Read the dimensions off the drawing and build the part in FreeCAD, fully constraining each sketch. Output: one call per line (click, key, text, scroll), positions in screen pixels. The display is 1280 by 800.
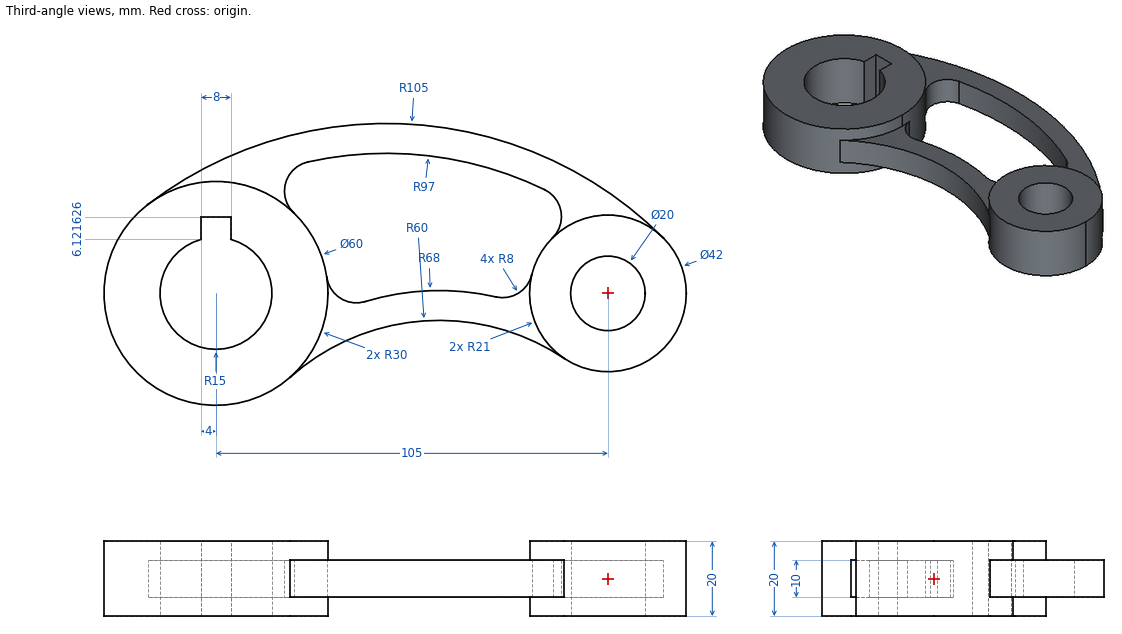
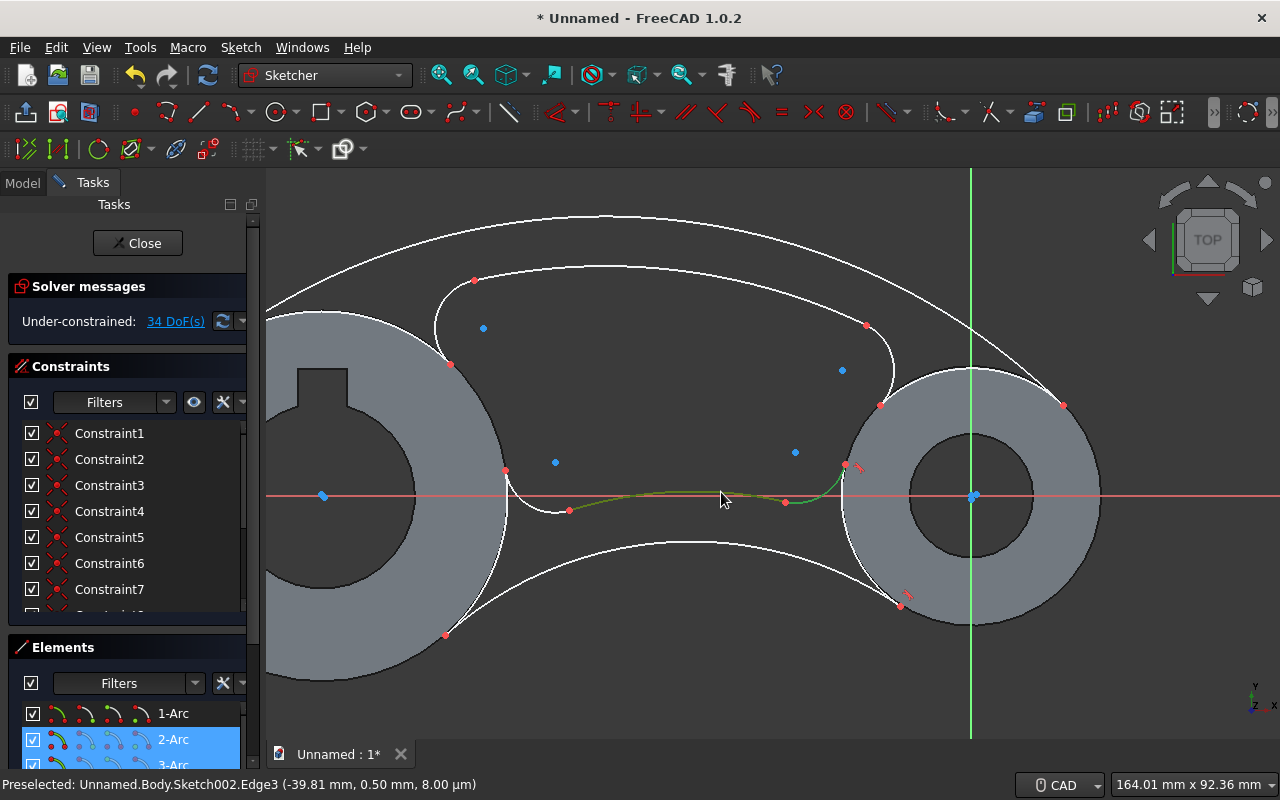
key(t)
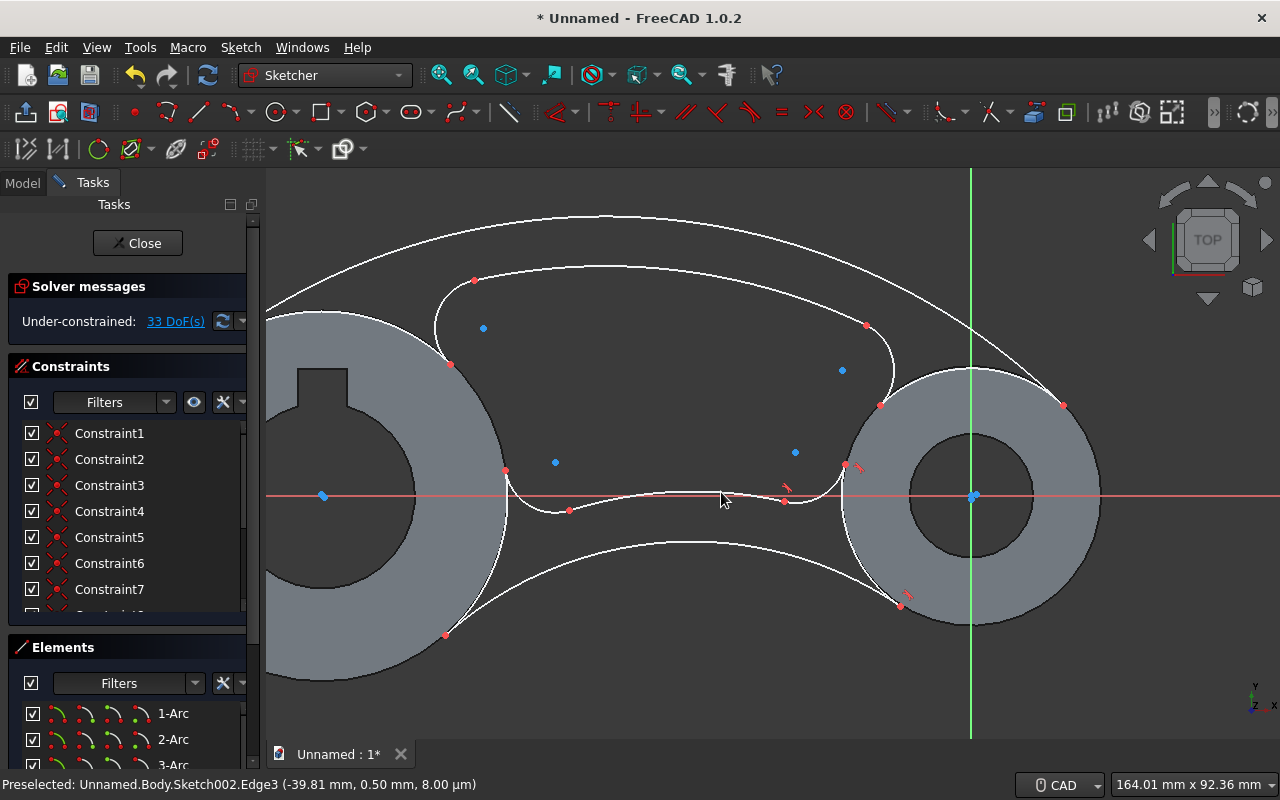
click(720, 492)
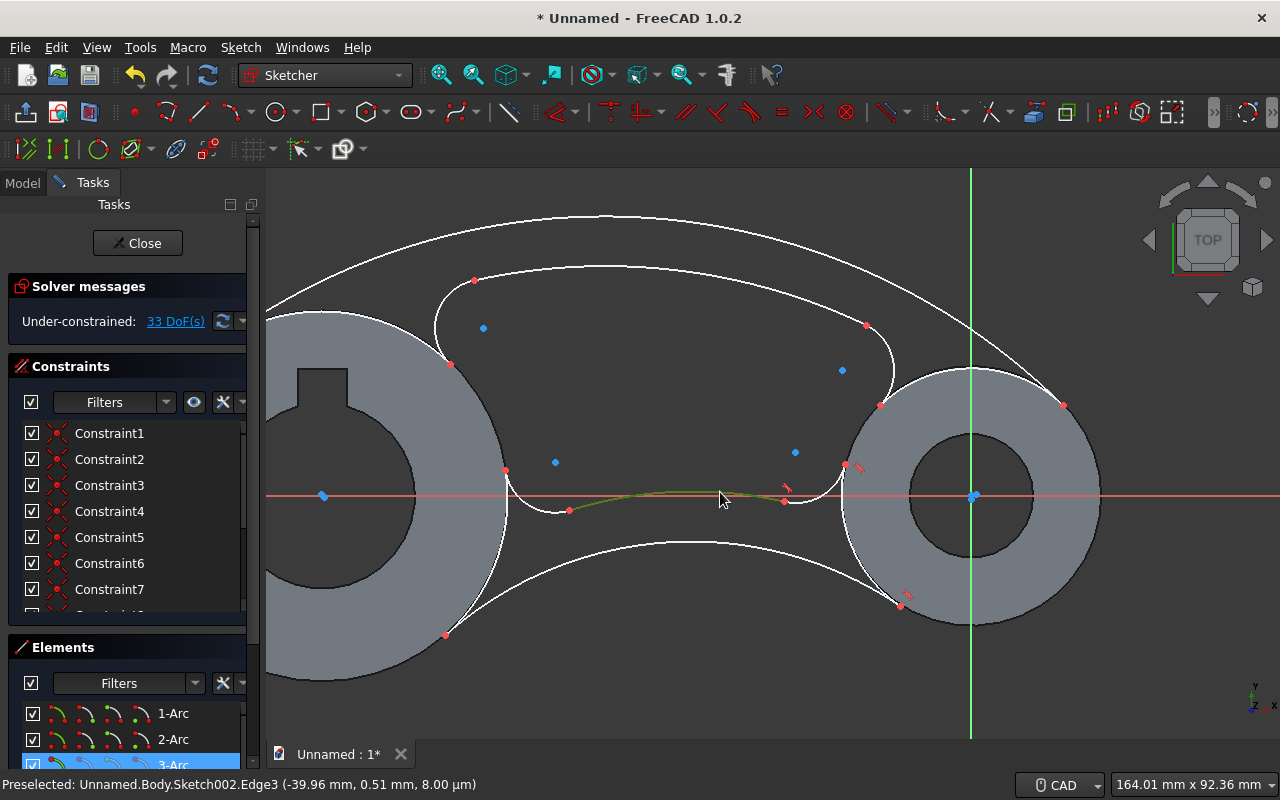
click(544, 511)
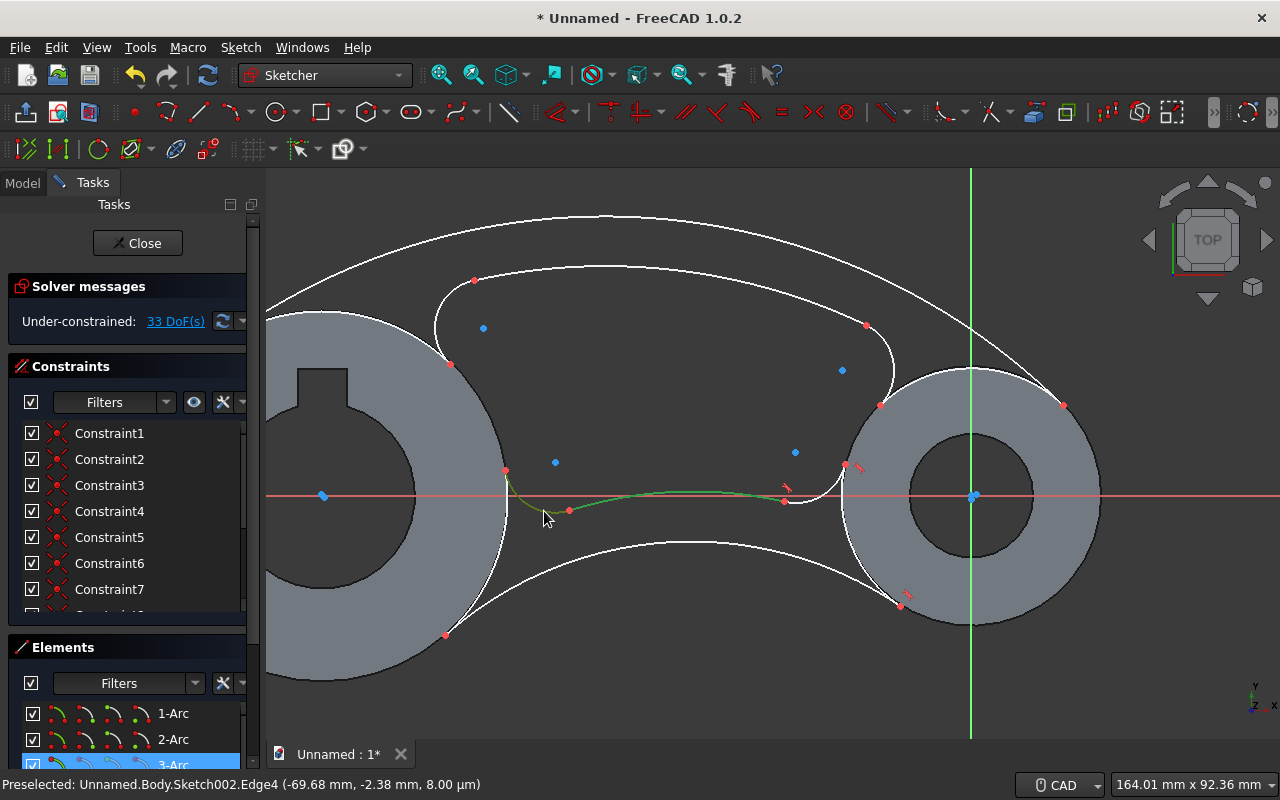
key(t)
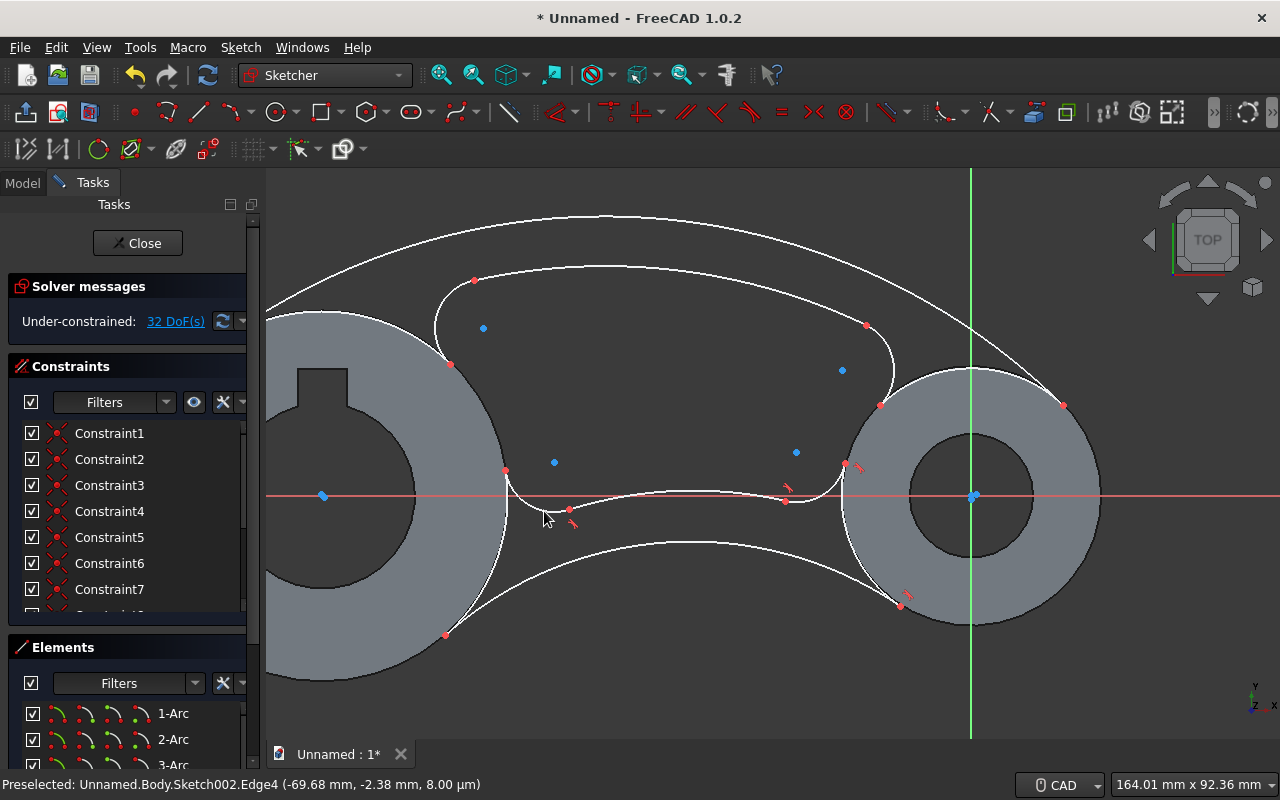
click(544, 511)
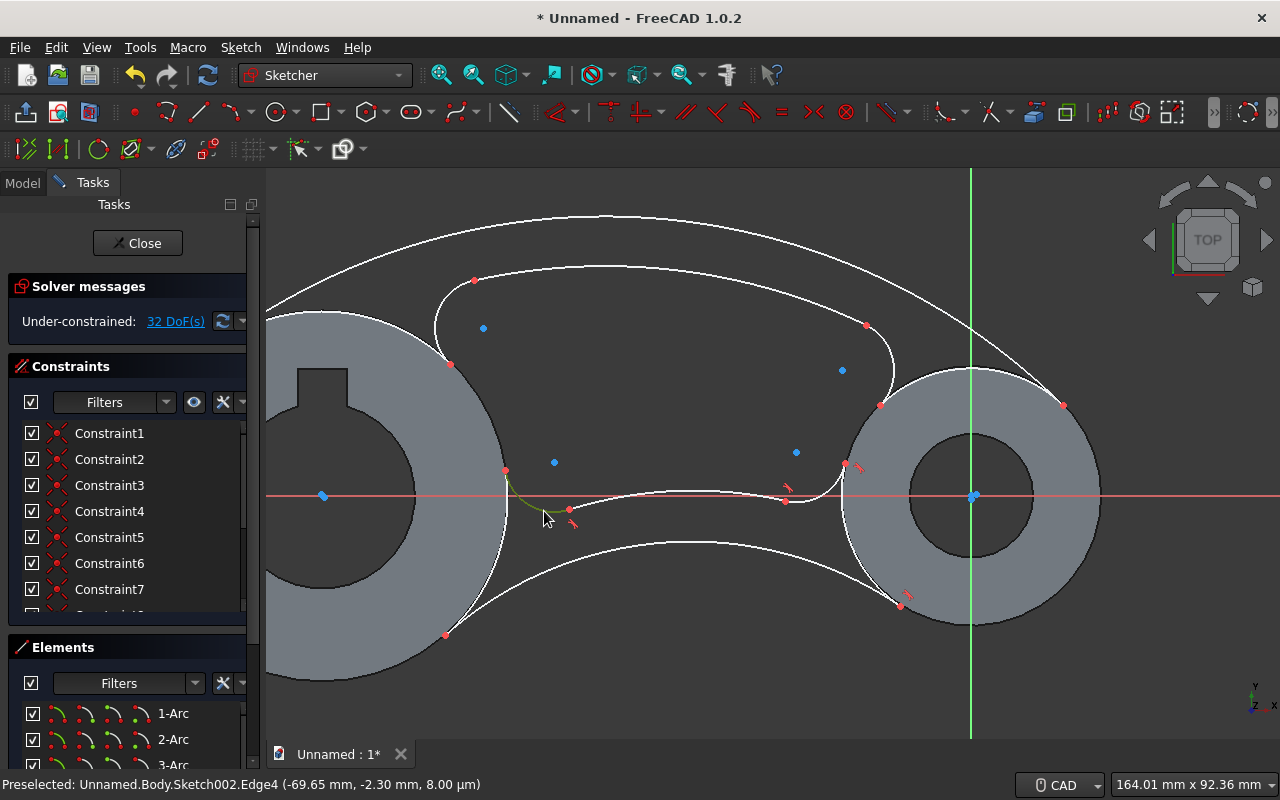
click(481, 593)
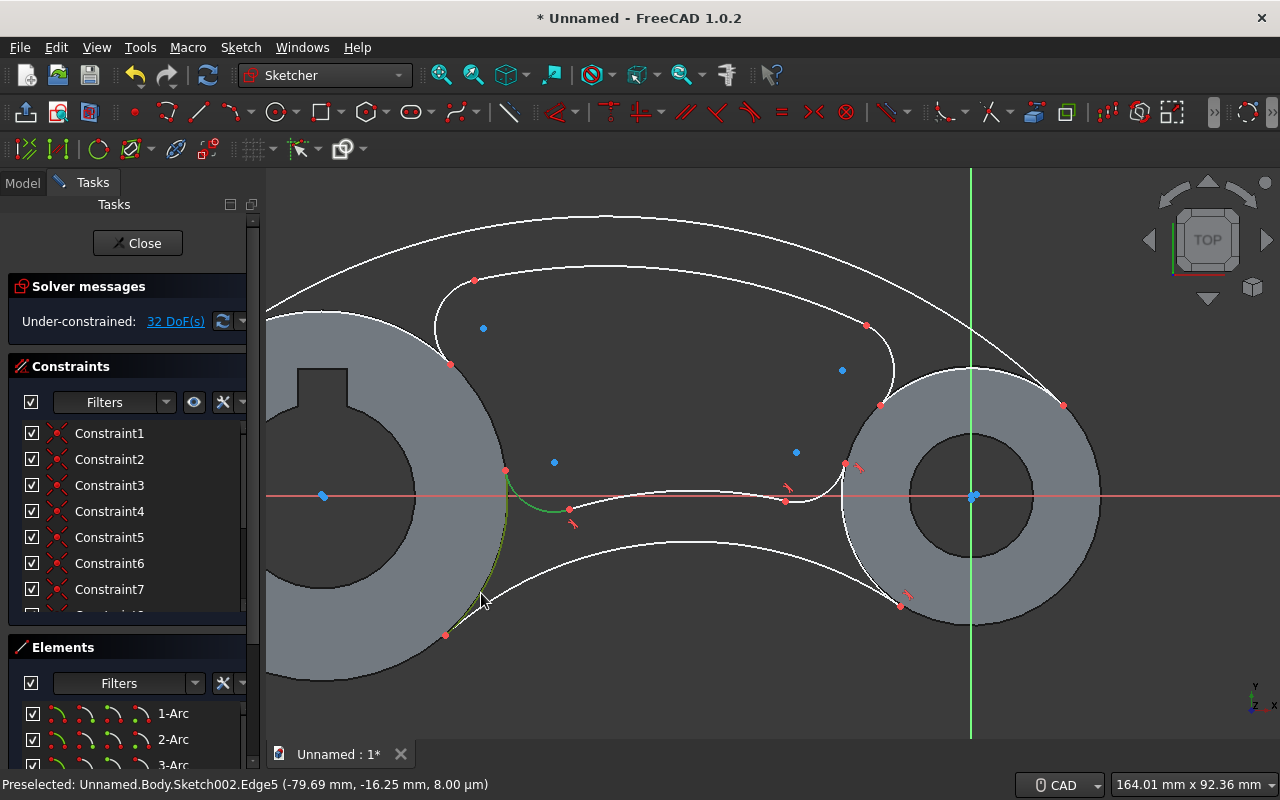
key(t)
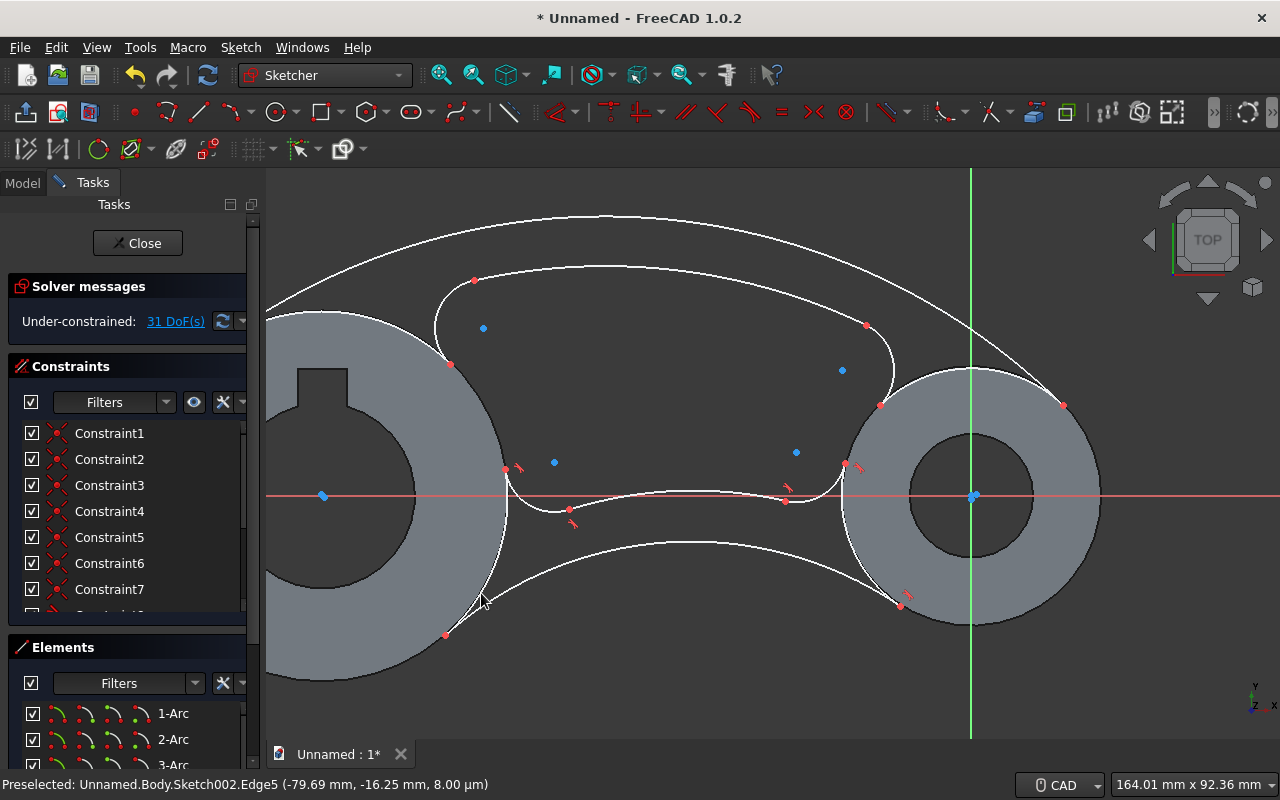
click(481, 593)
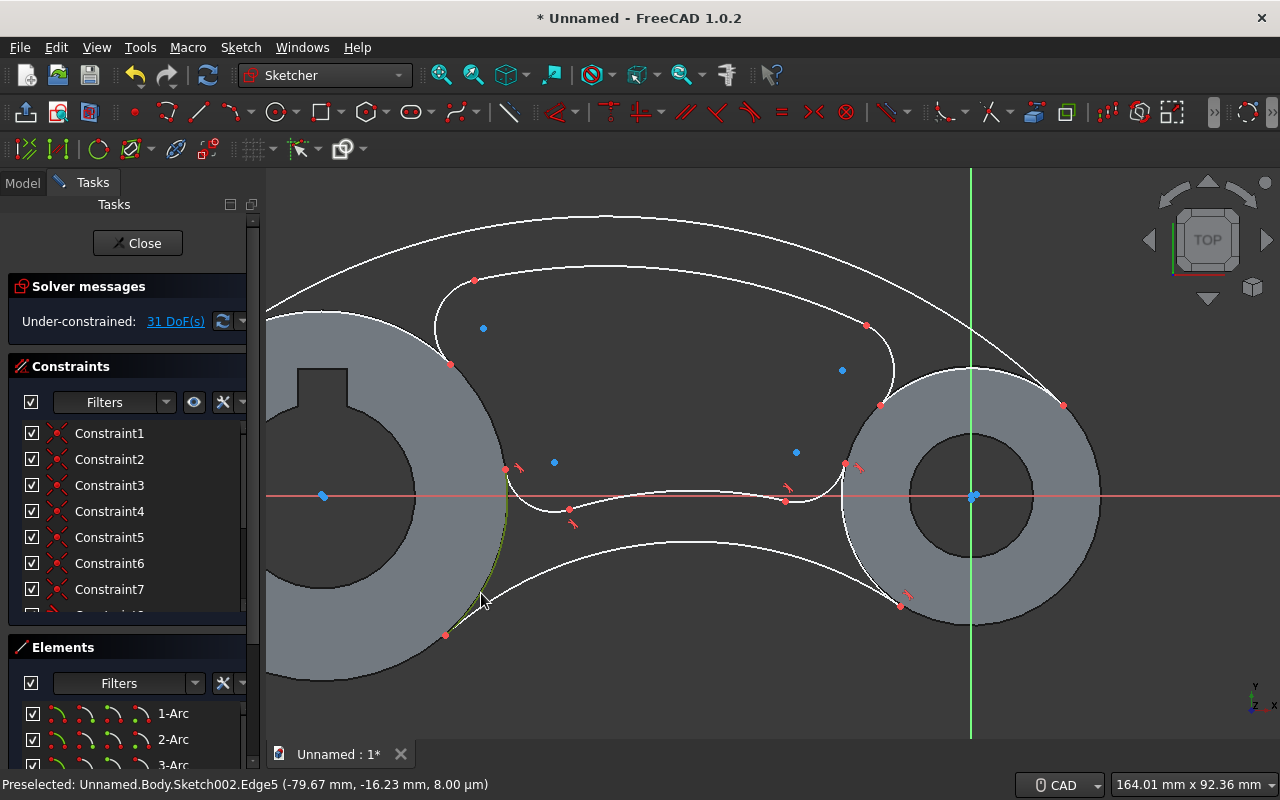
click(766, 549)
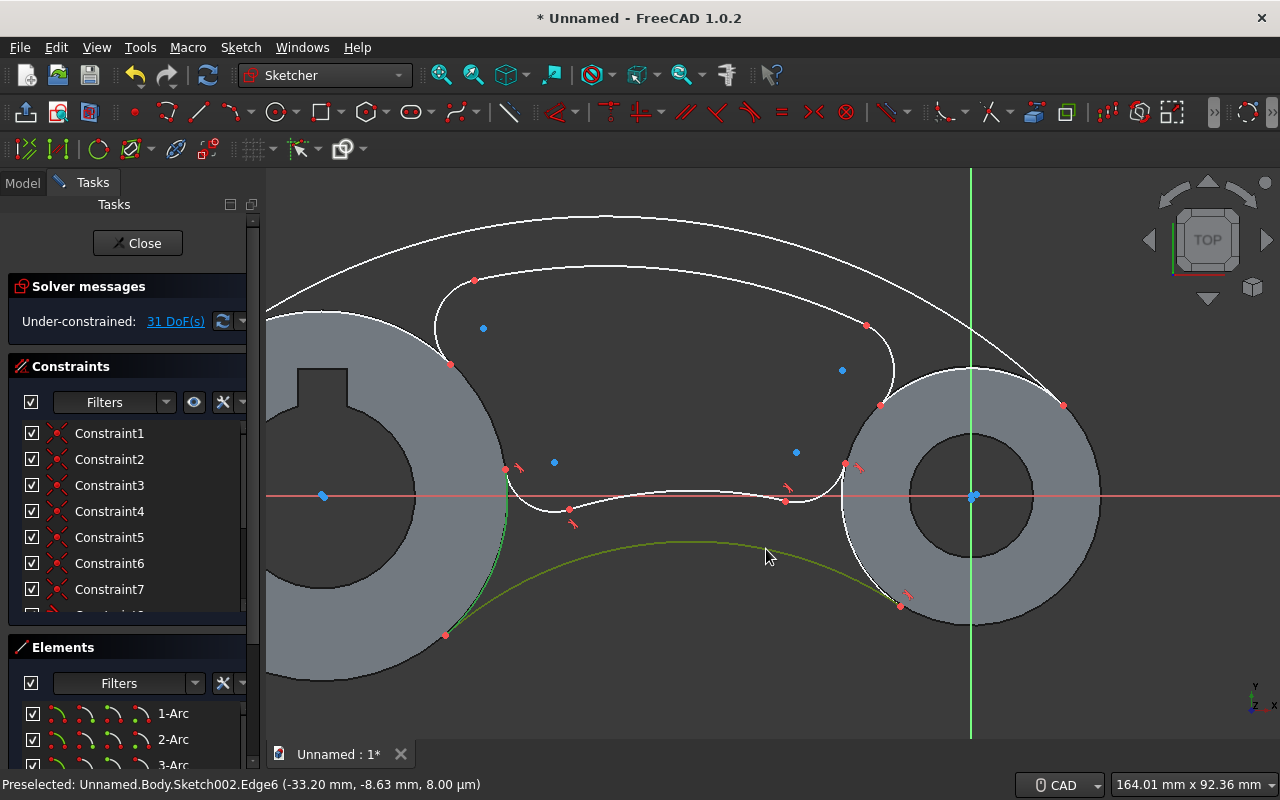
key(t)